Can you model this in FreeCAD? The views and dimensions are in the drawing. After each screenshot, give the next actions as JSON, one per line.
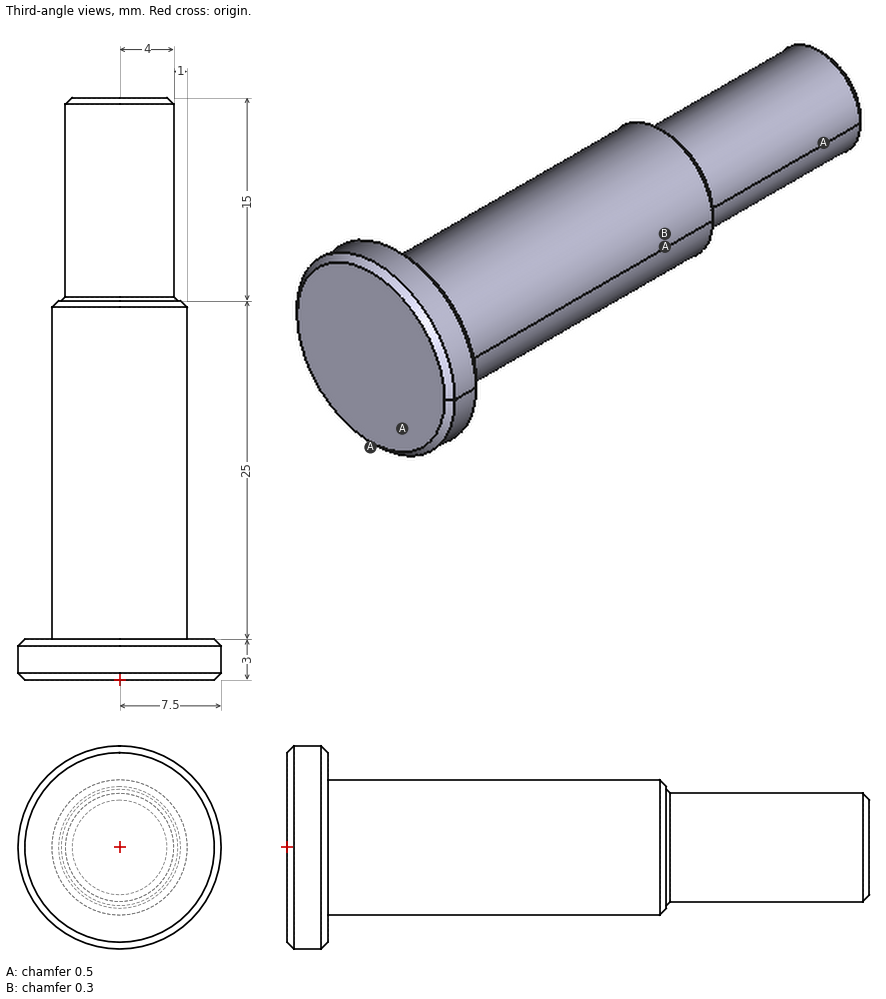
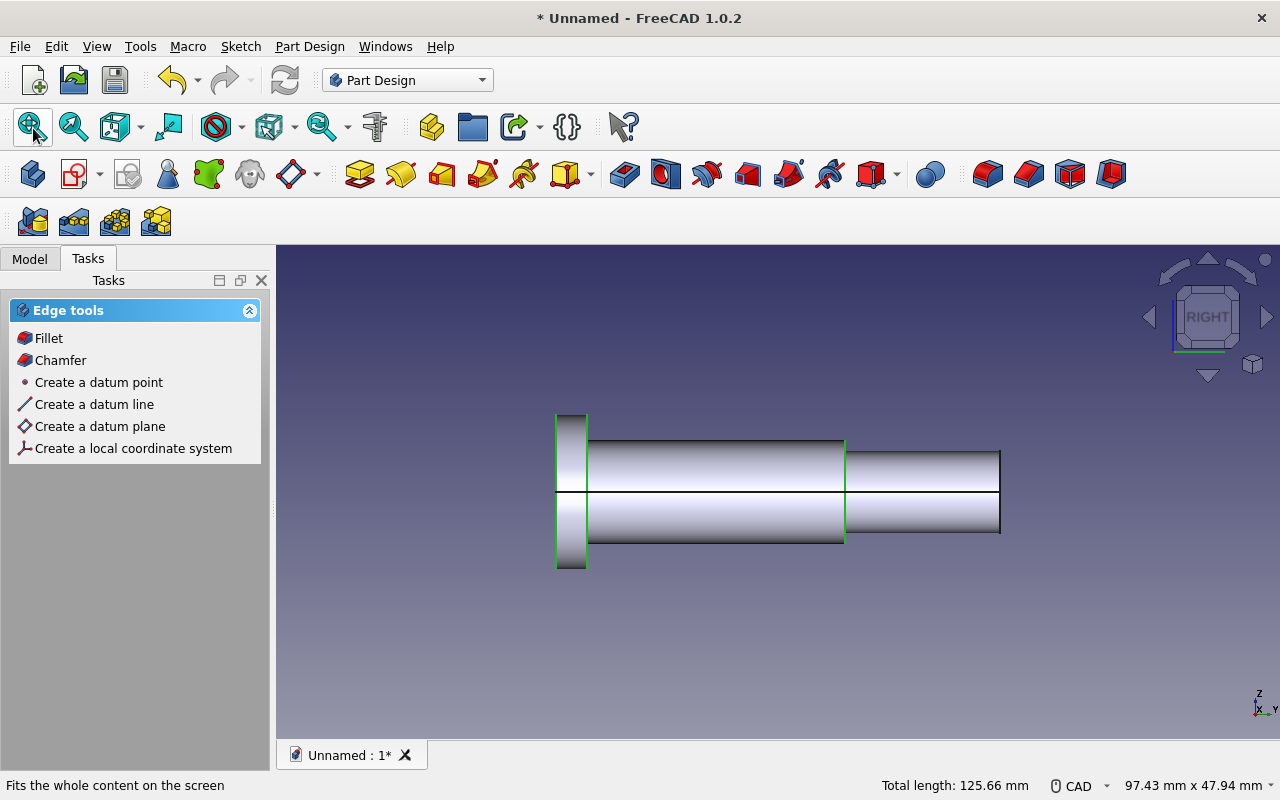
{"action": "left_click", "coordinate": [33, 128]}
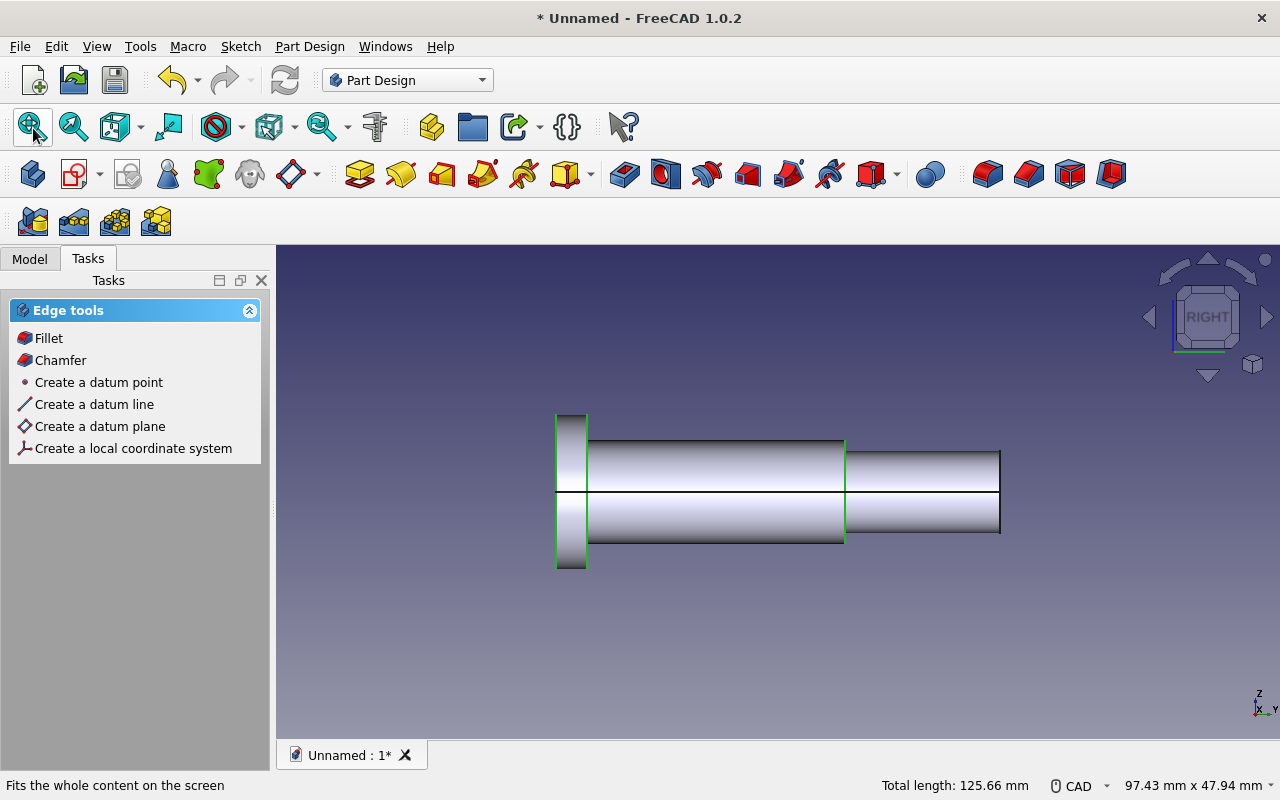
{"action": "left_click", "coordinate": [1000, 467], "text": "ctrl"}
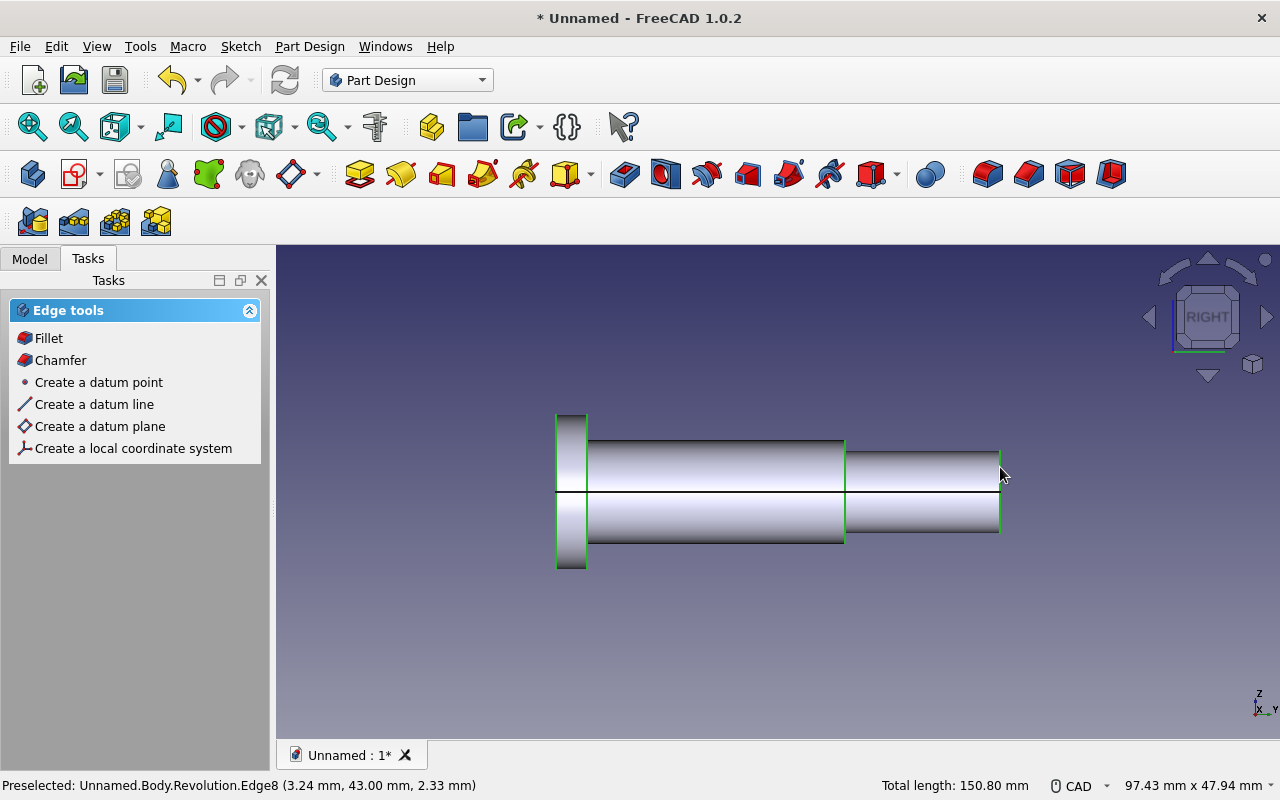
{"action": "left_click", "coordinate": [1029, 174]}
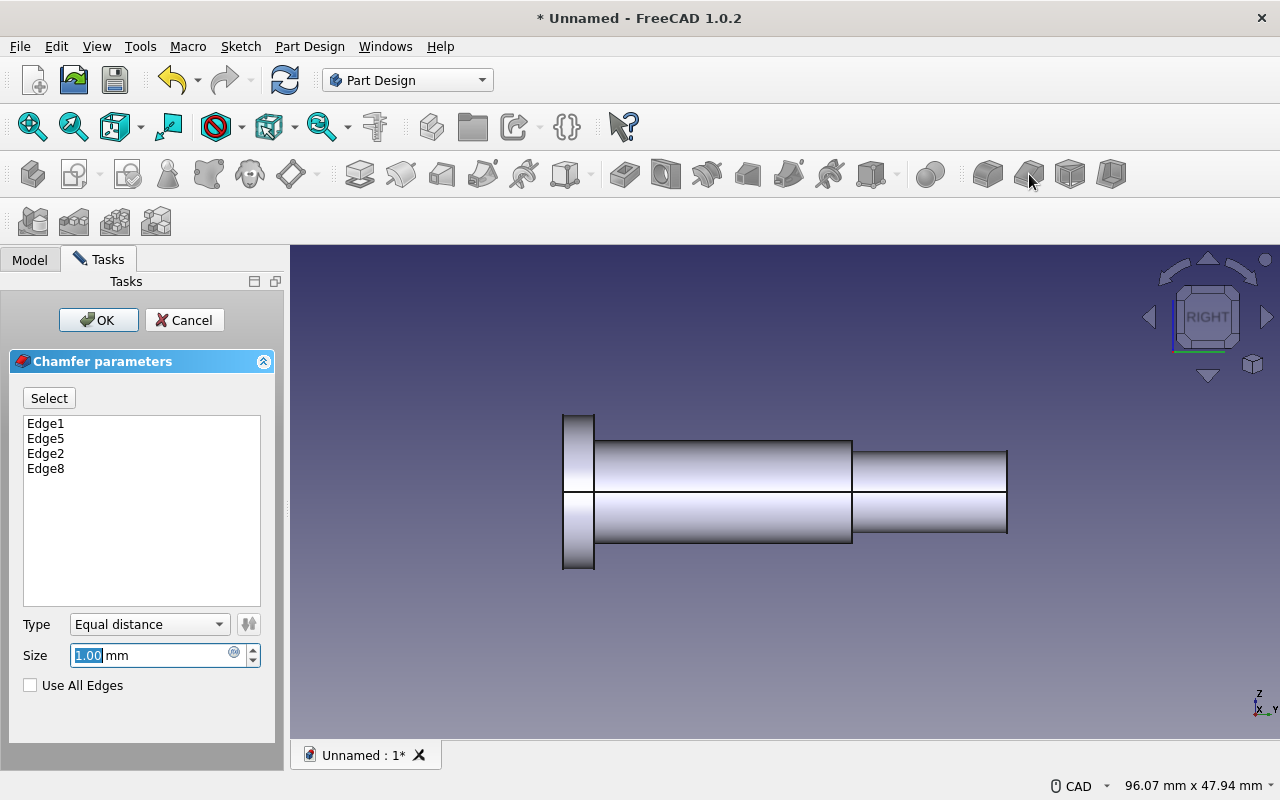
{"action": "type", "text": "0.5"}
{"action": "key", "text": "Tab"}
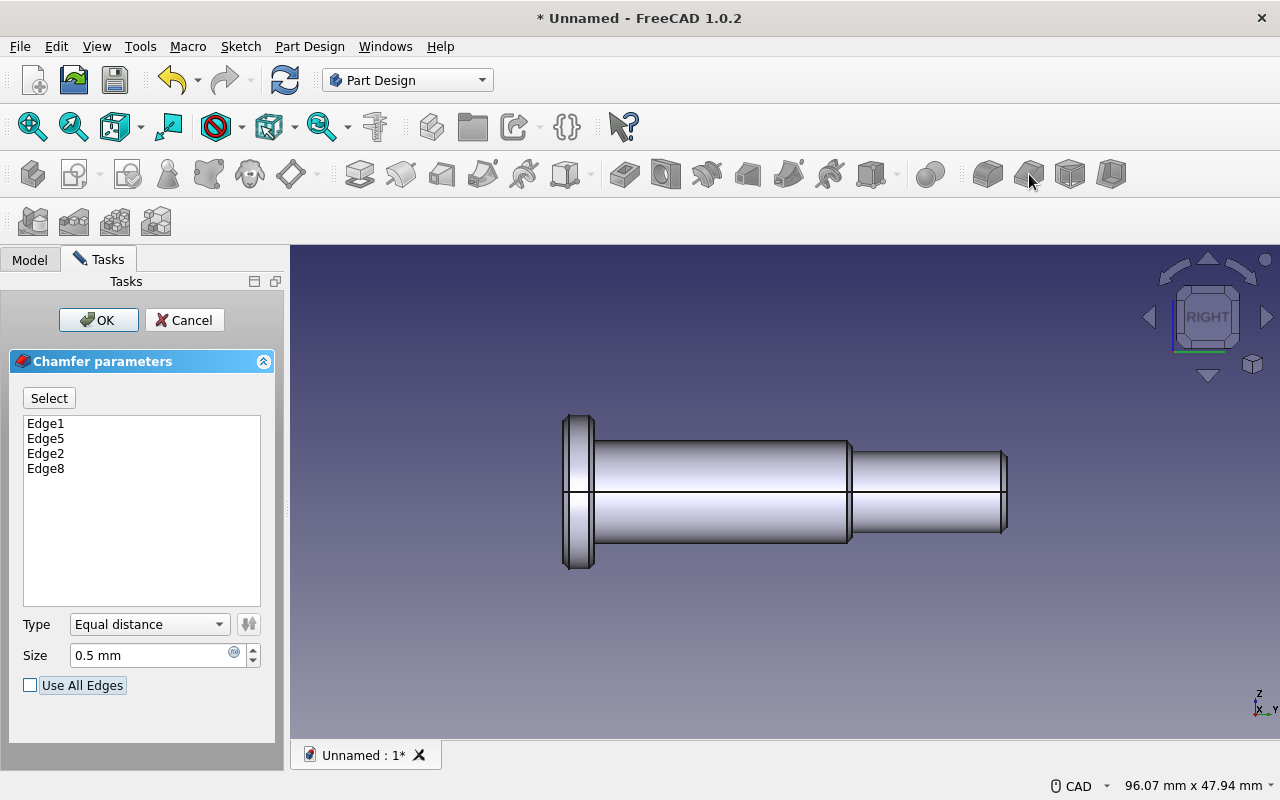
{"action": "left_click", "coordinate": [99, 320]}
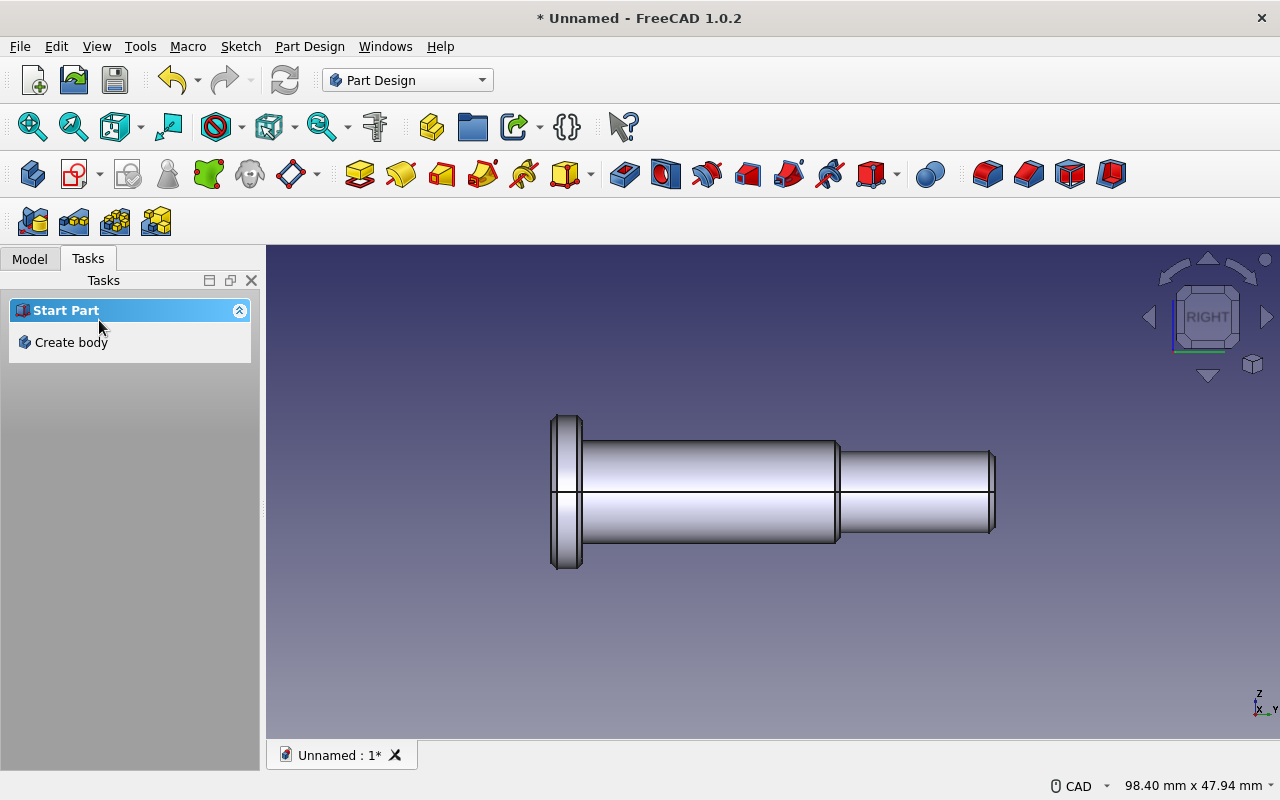
{"action": "left_click", "coordinate": [33, 128]}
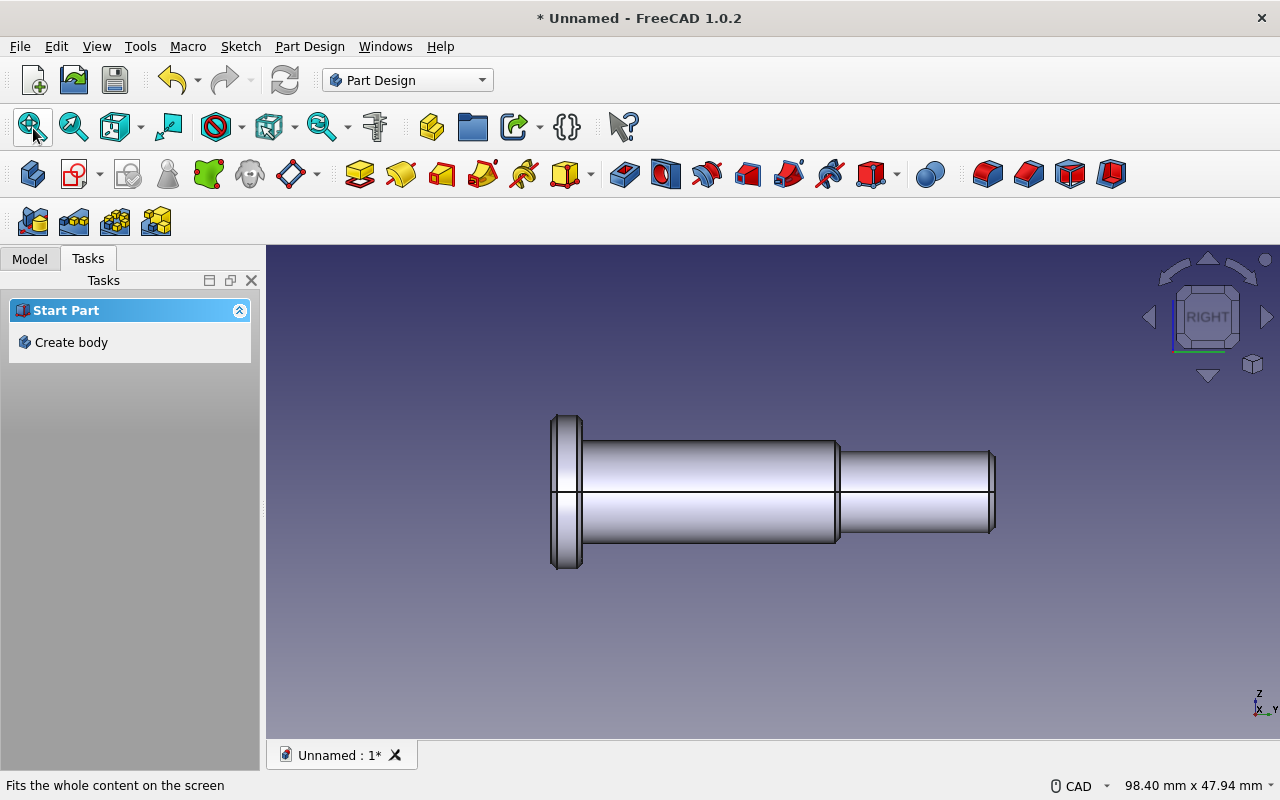
{"action": "key", "text": "0"}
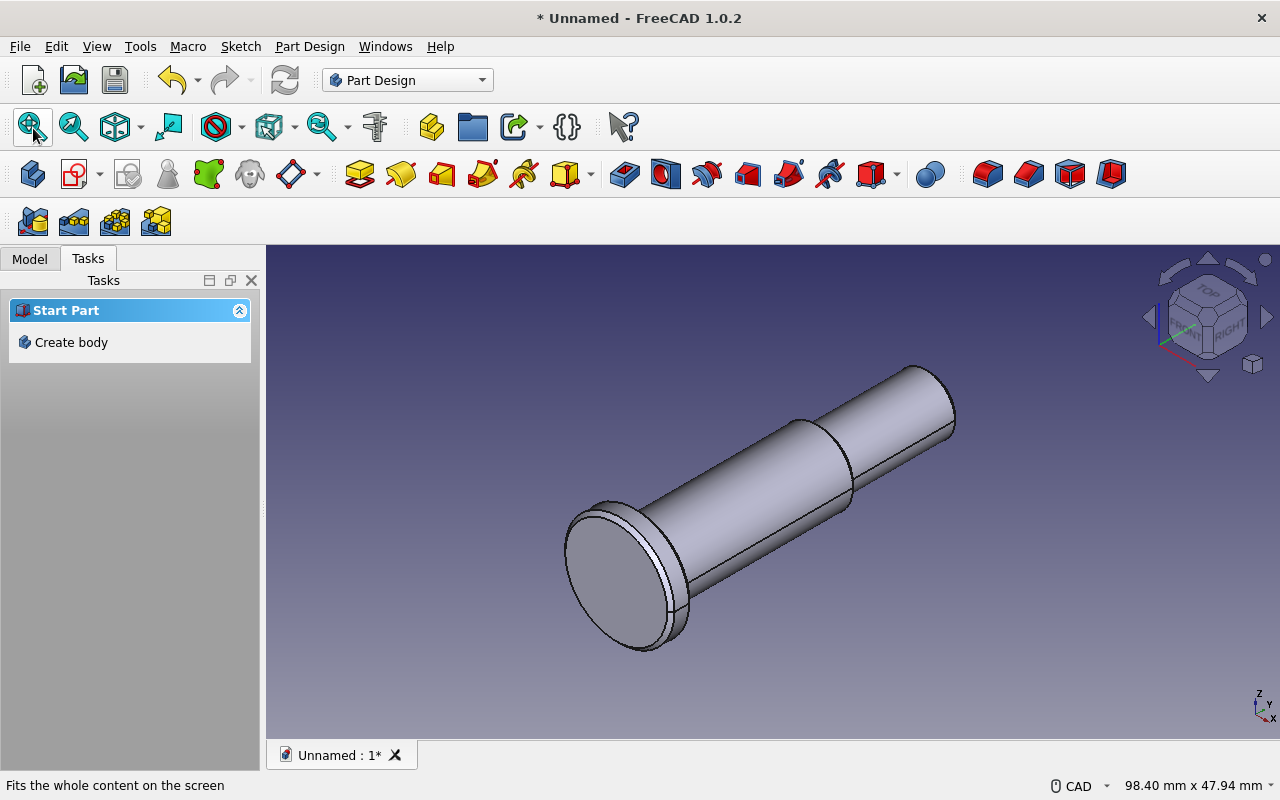
{"action": "key", "text": "2"}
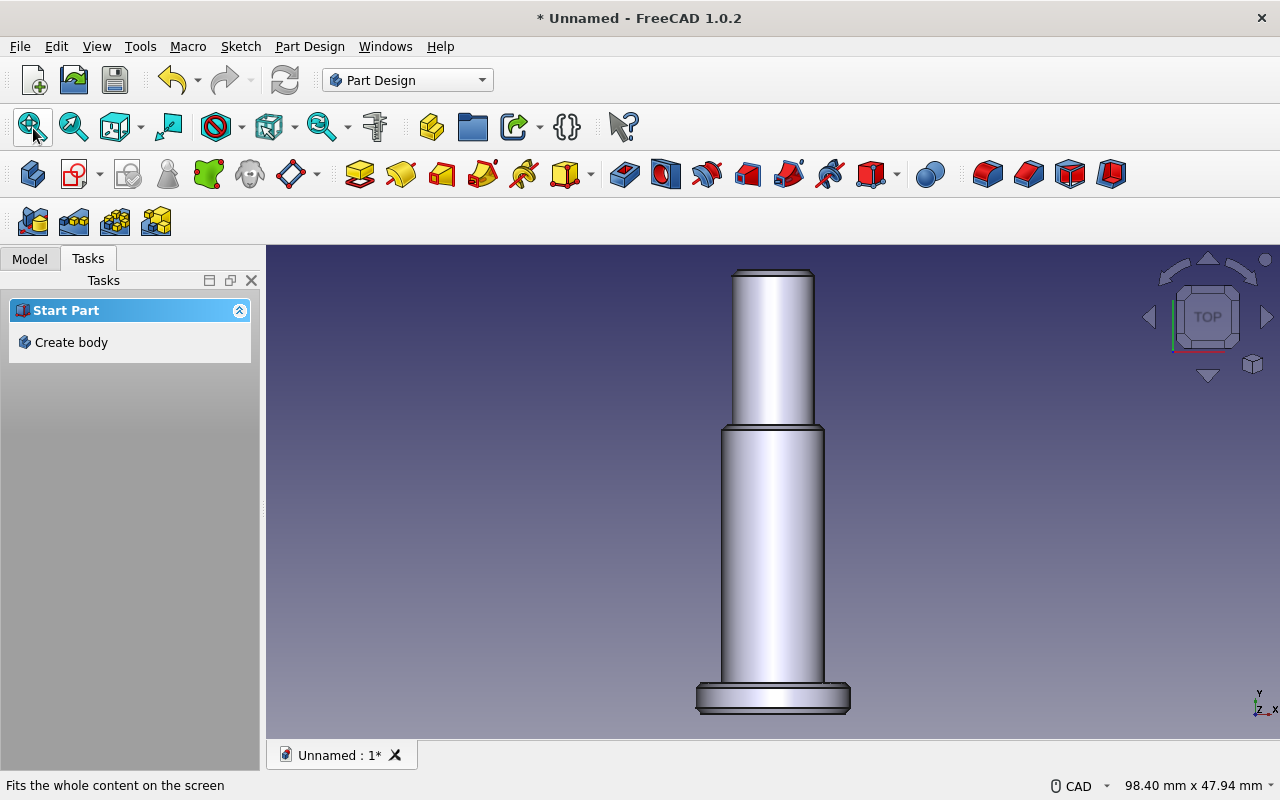
{"action": "key", "text": "1"}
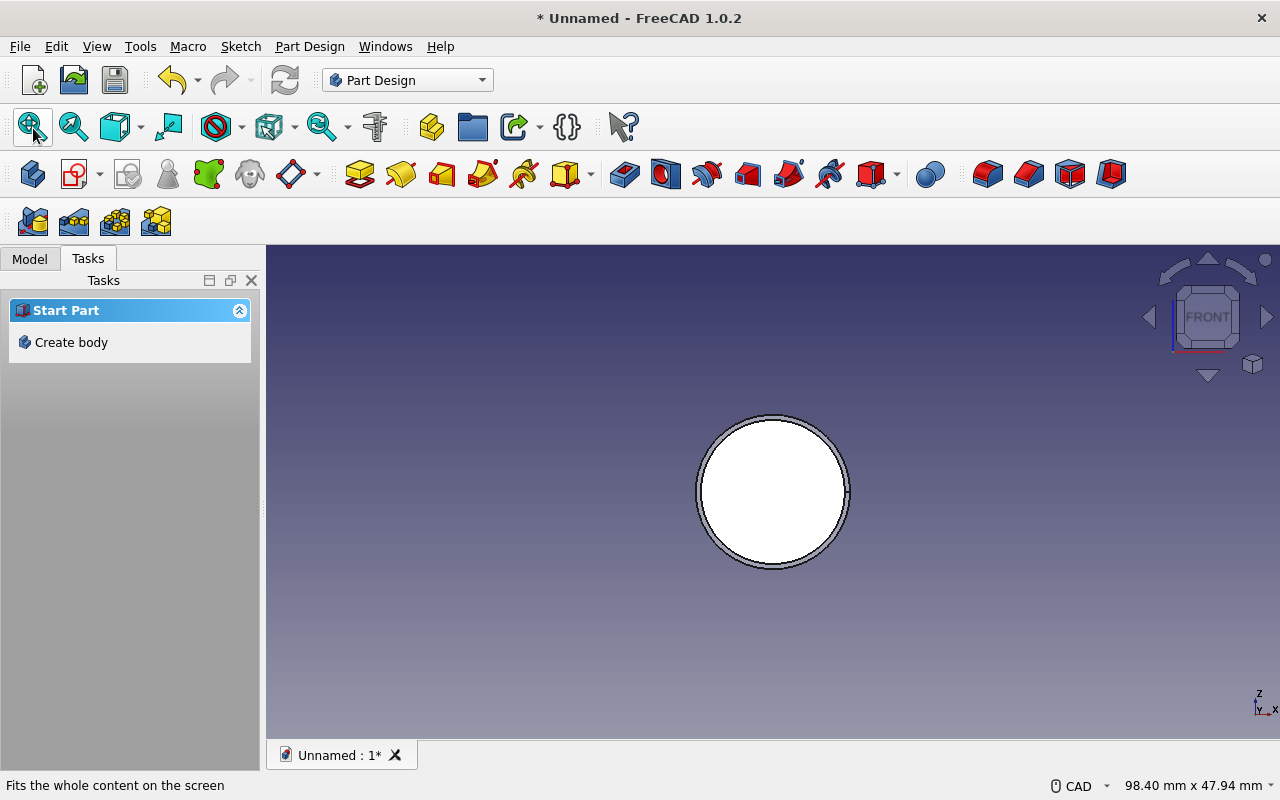
{"action": "left_click", "coordinate": [33, 128]}